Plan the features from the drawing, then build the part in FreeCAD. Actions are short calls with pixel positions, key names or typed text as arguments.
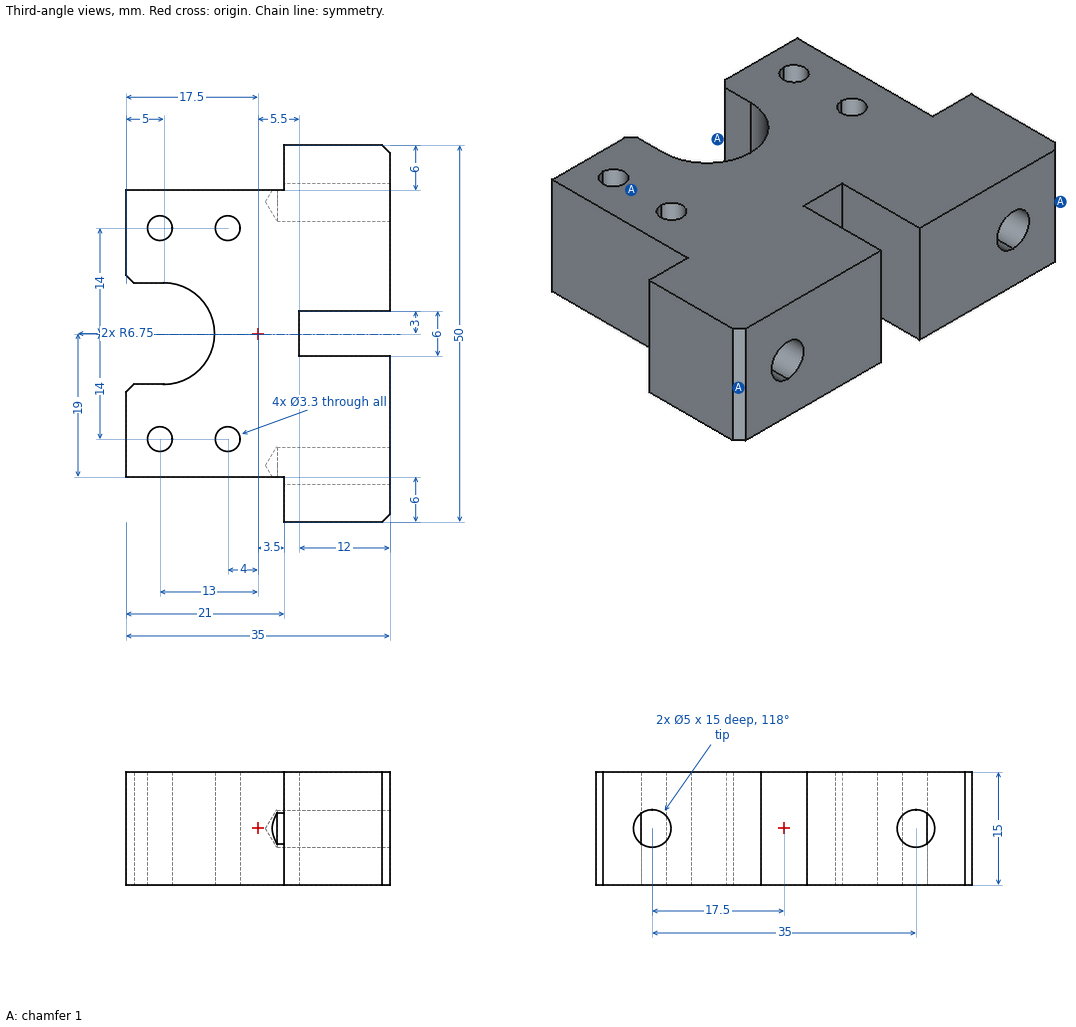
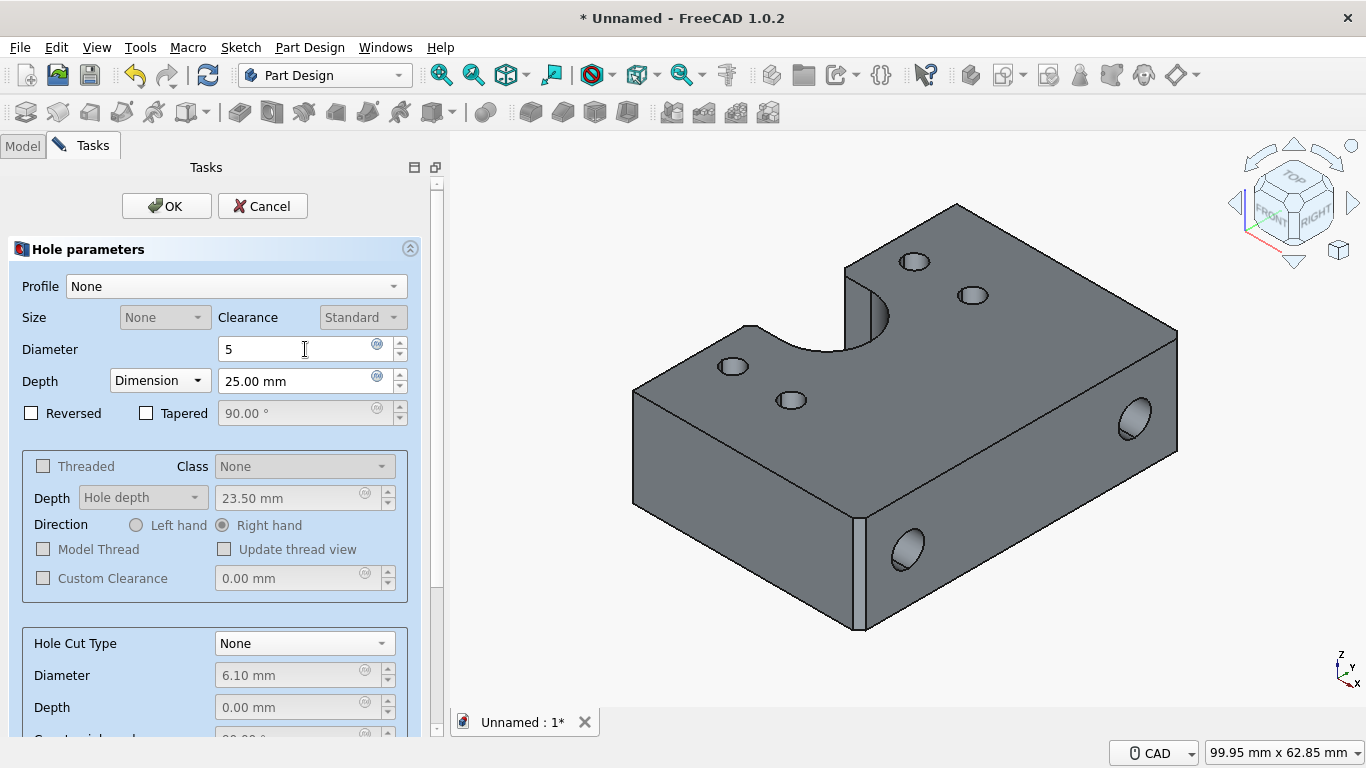
triple_click(305, 381)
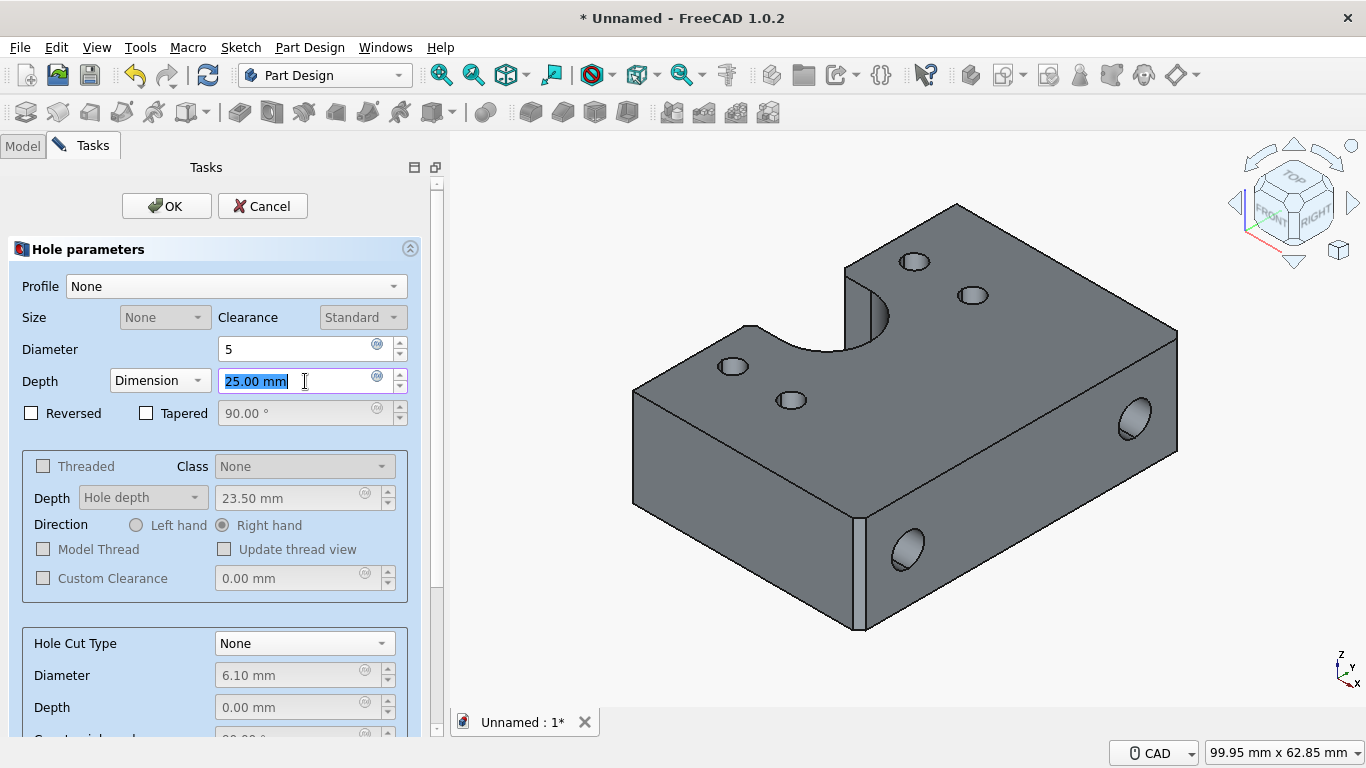
text(15)
key(Tab)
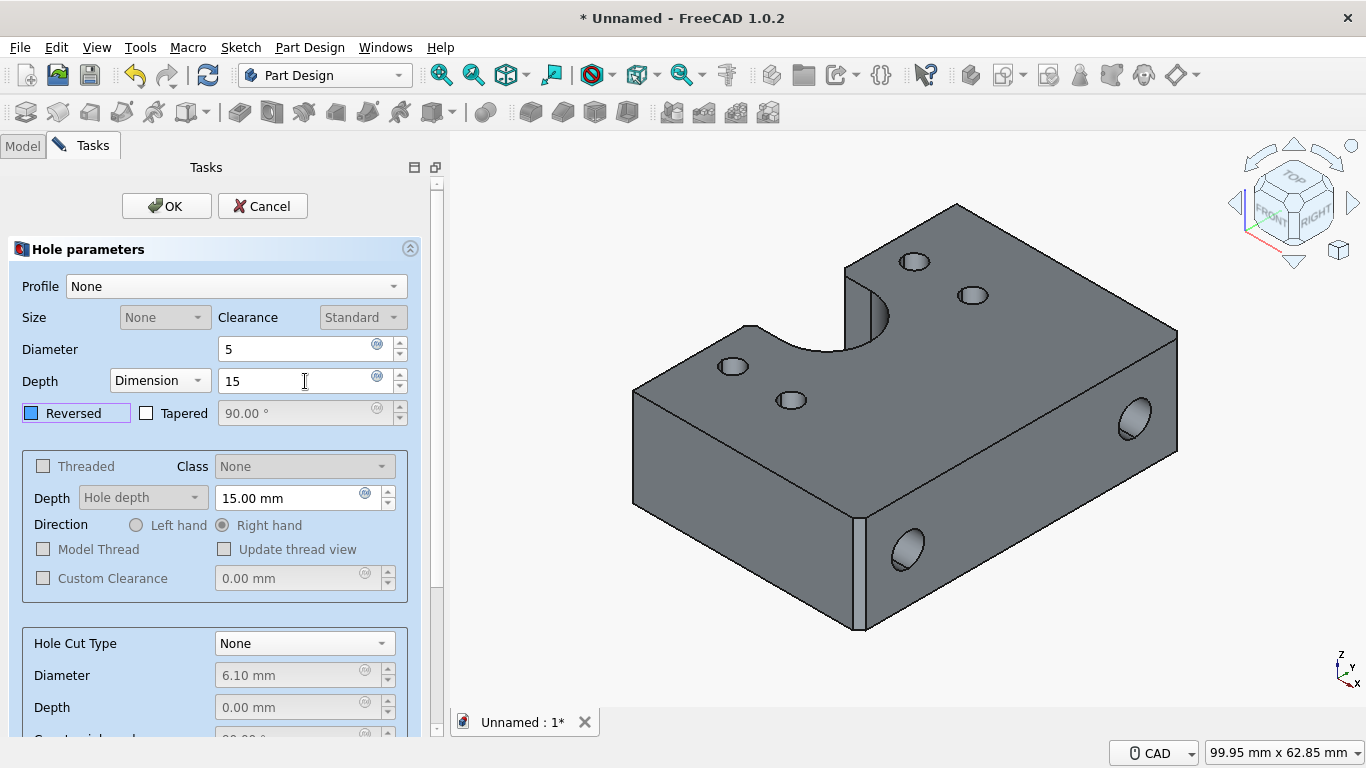
click(167, 206)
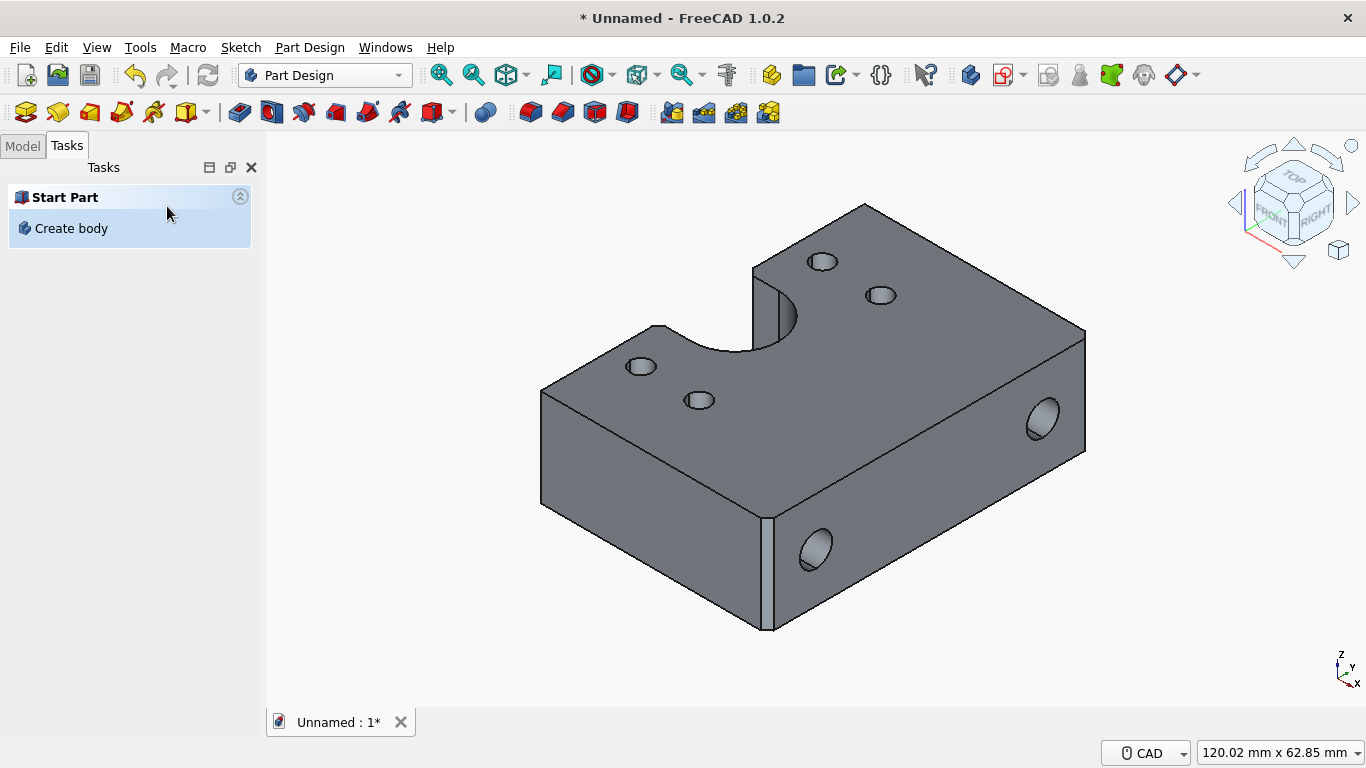
click(848, 381)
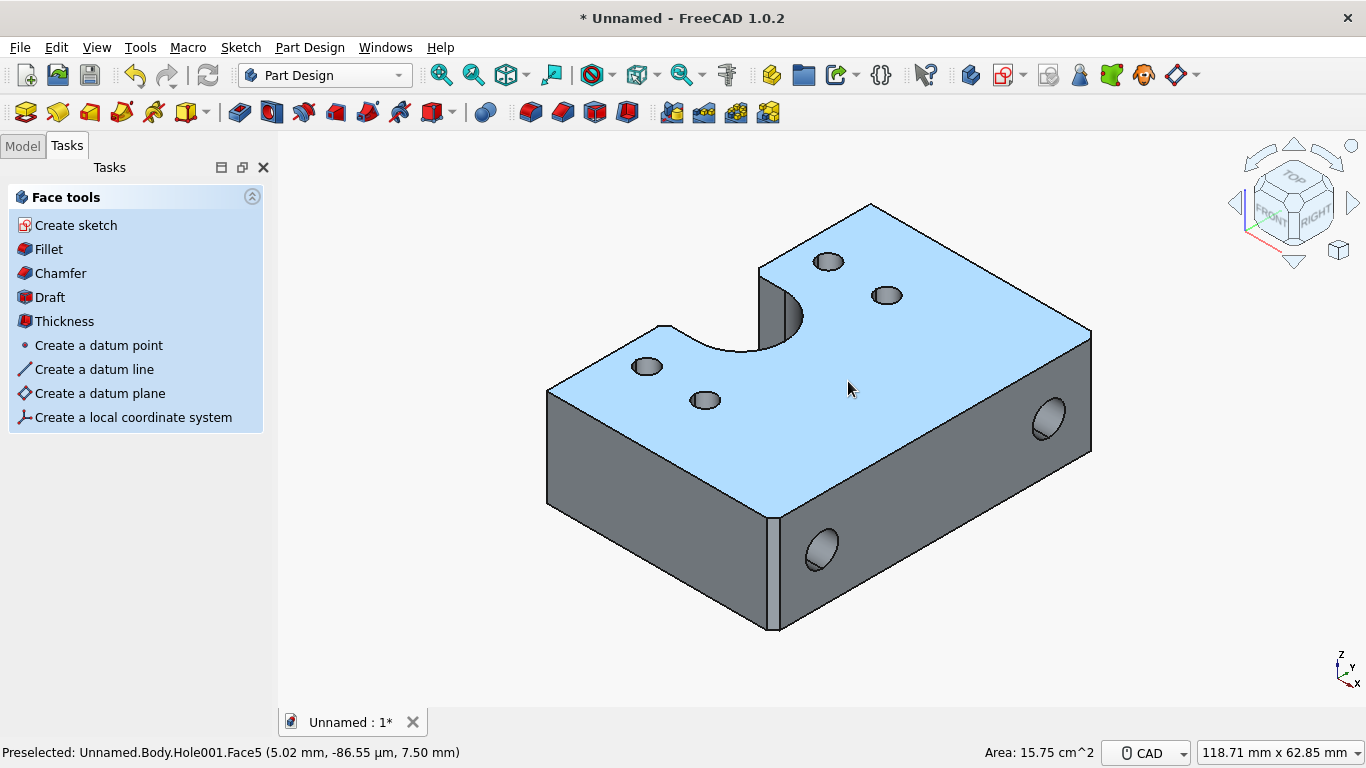
click(1004, 76)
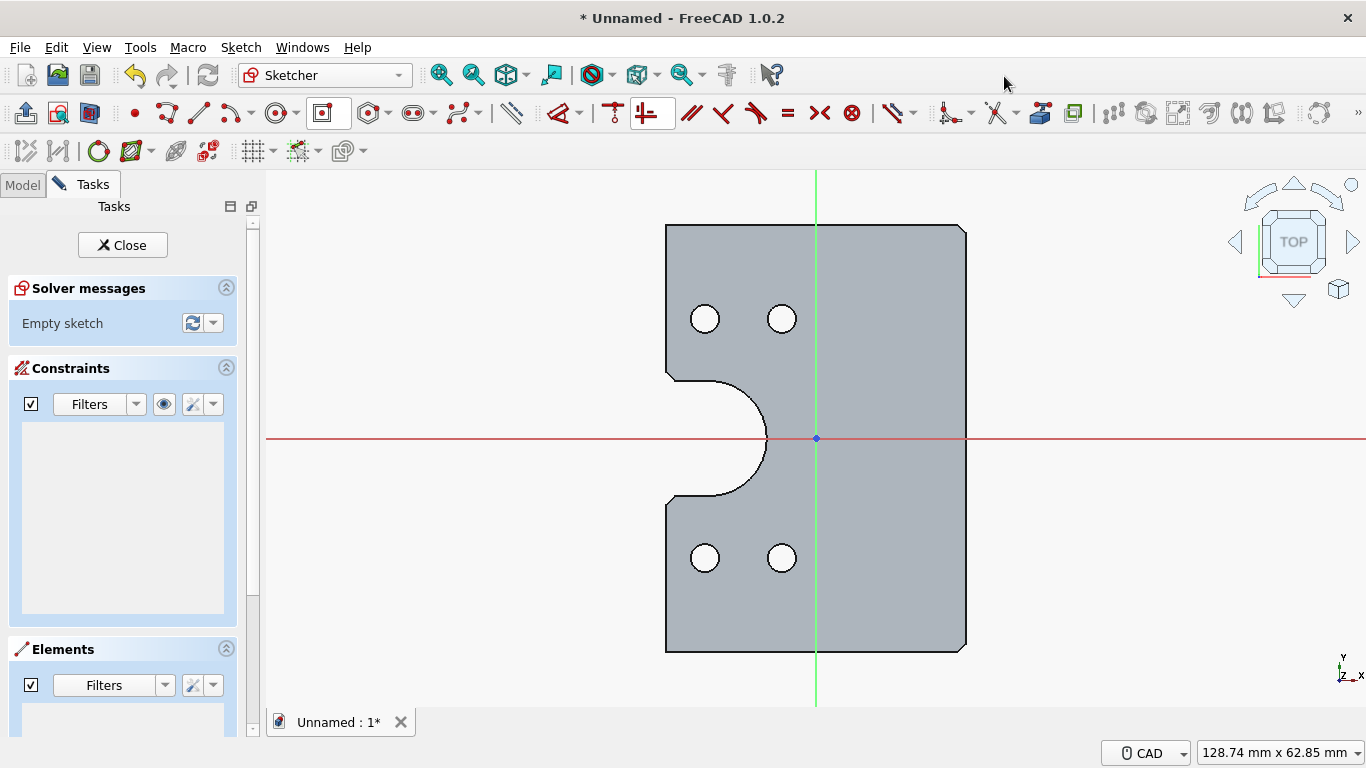
scroll(938, 438, up, 7)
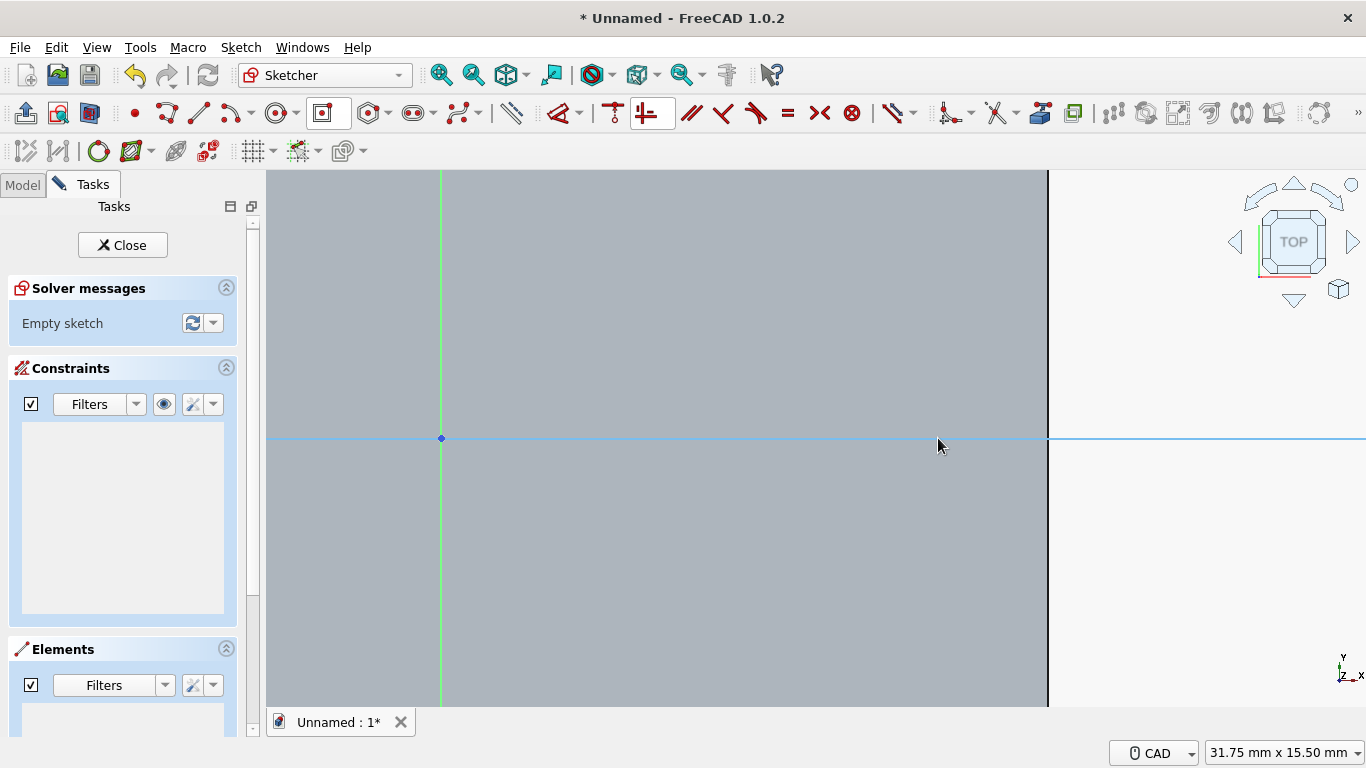
key(g)
key(r)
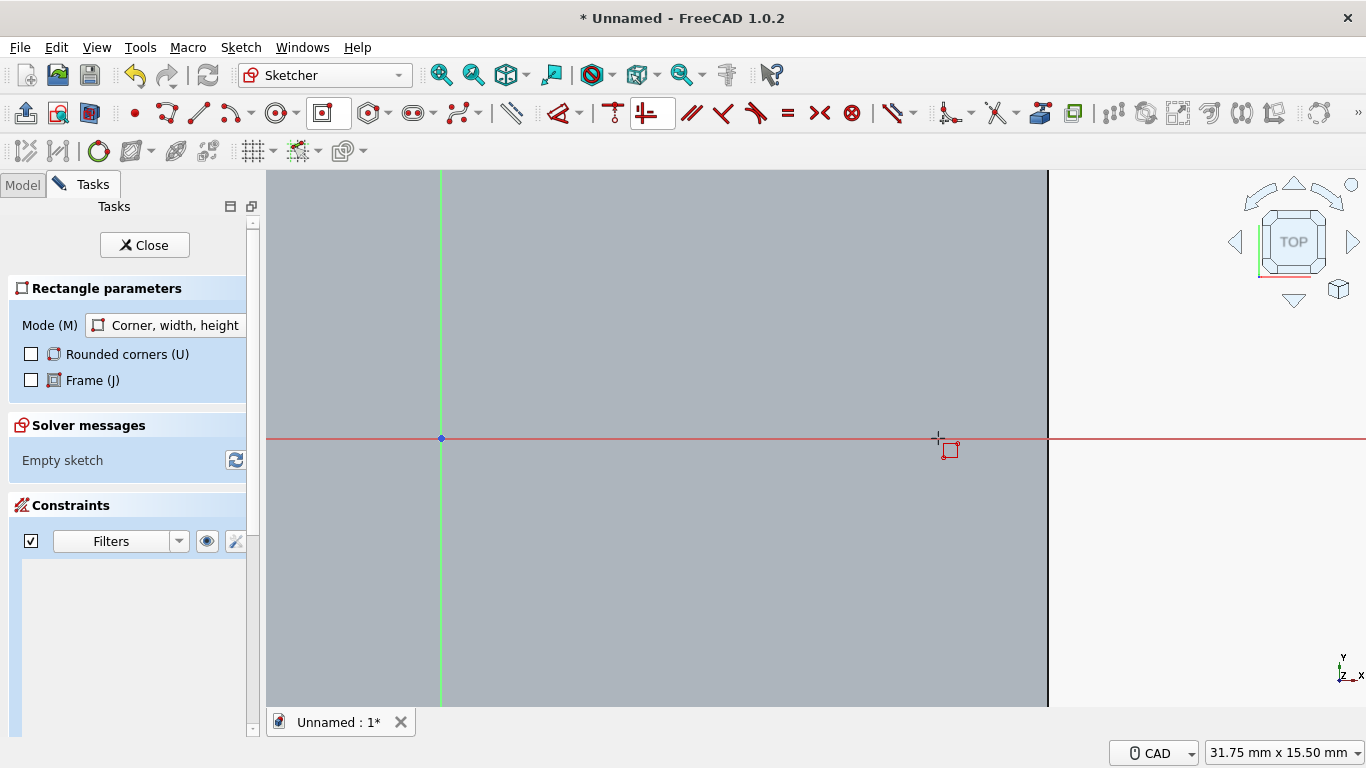
click(632, 335)
move(1048, 542)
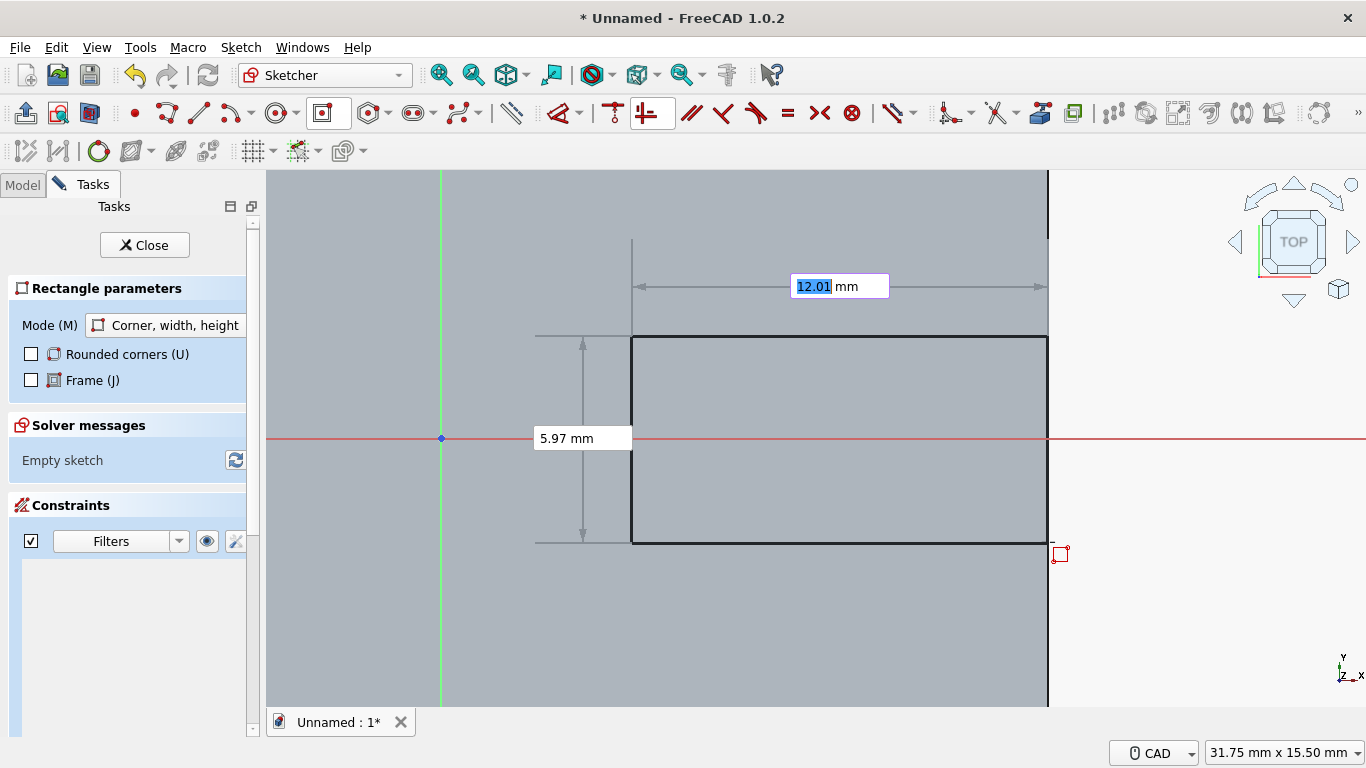
text(12)
key(Tab)
text(6)
key(Return)
key(Escape)